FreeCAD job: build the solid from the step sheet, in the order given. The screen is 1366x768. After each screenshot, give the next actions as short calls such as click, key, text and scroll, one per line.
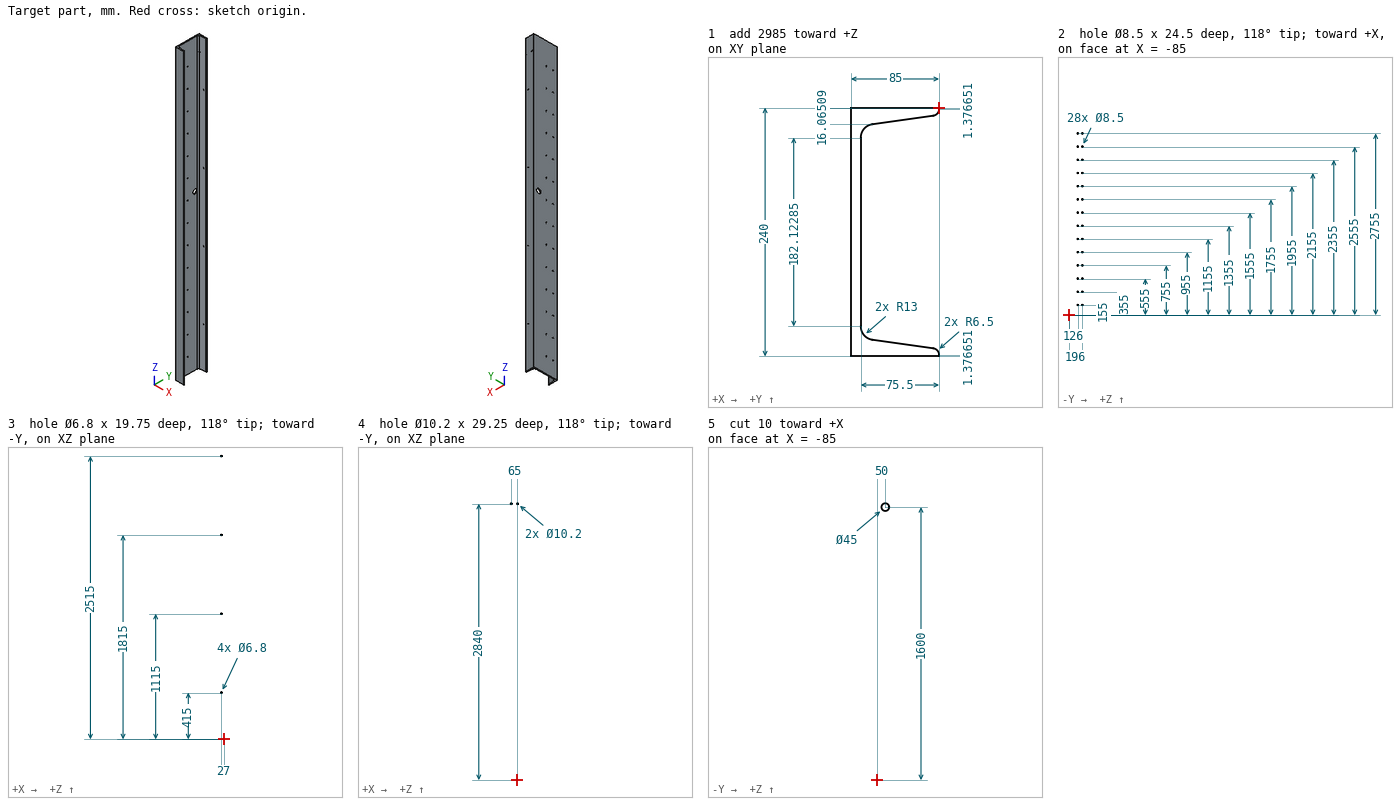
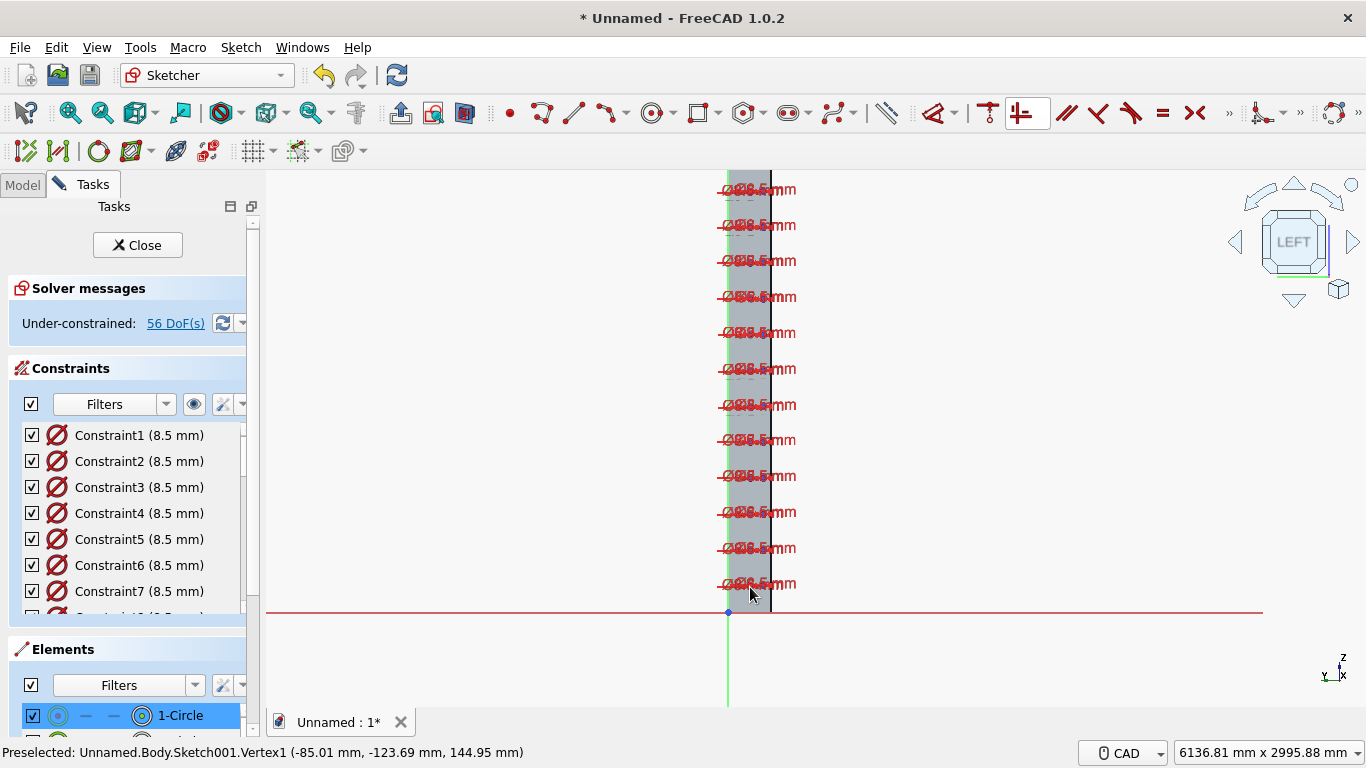
click(764, 585)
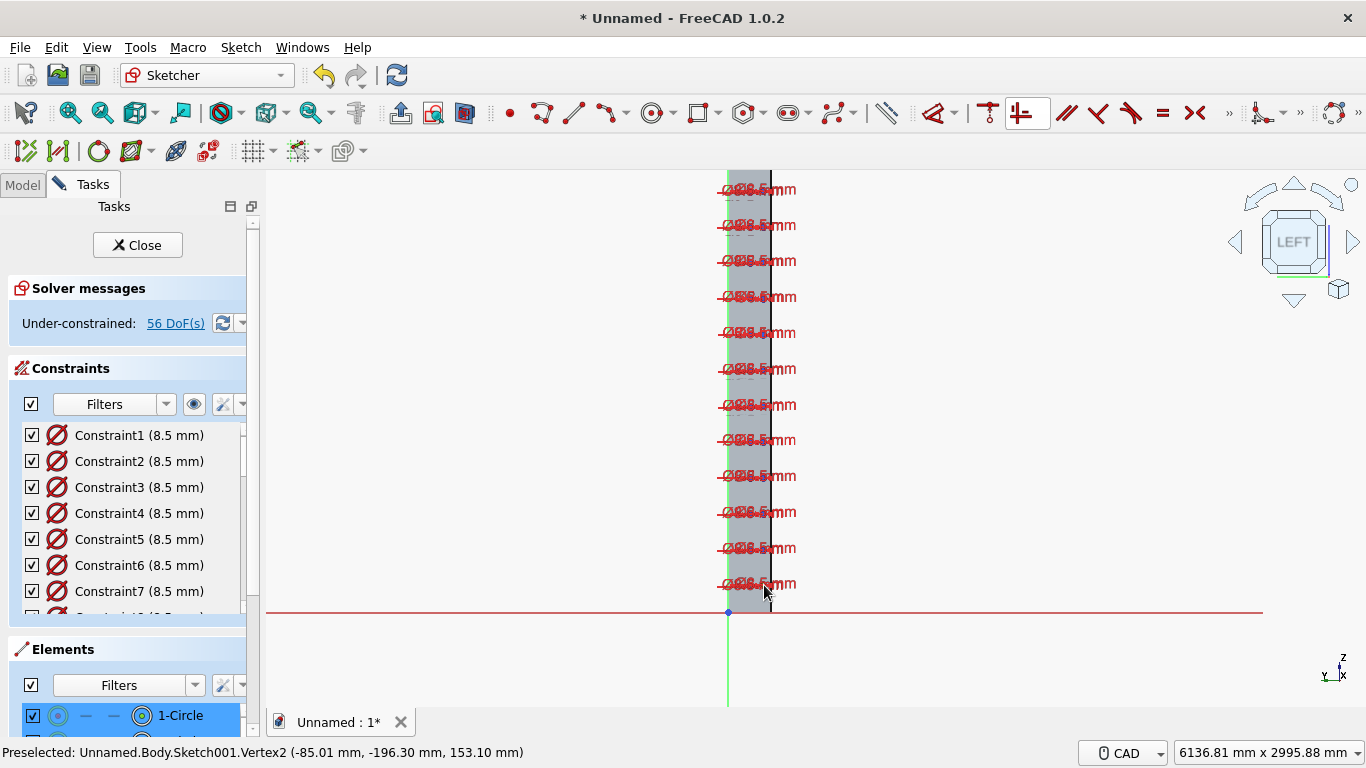
click(1044, 114)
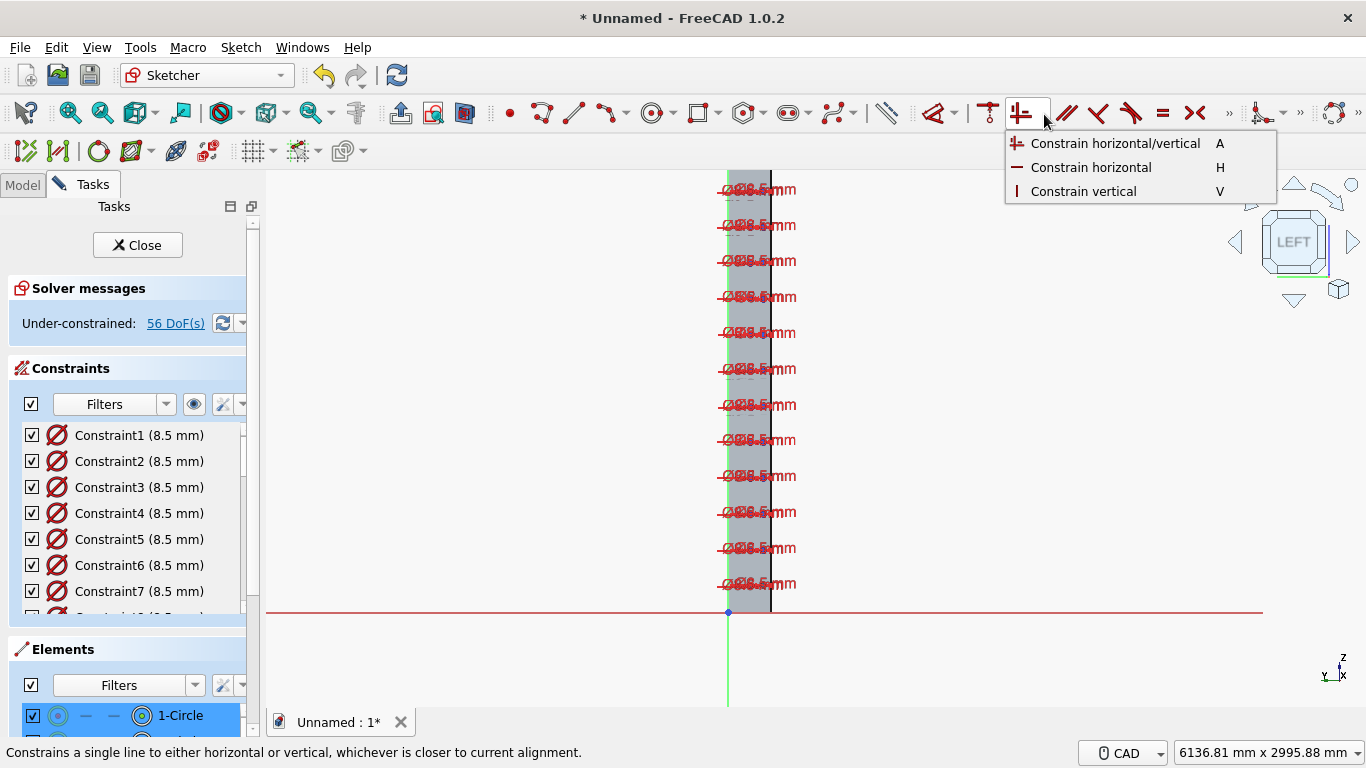
click(1141, 167)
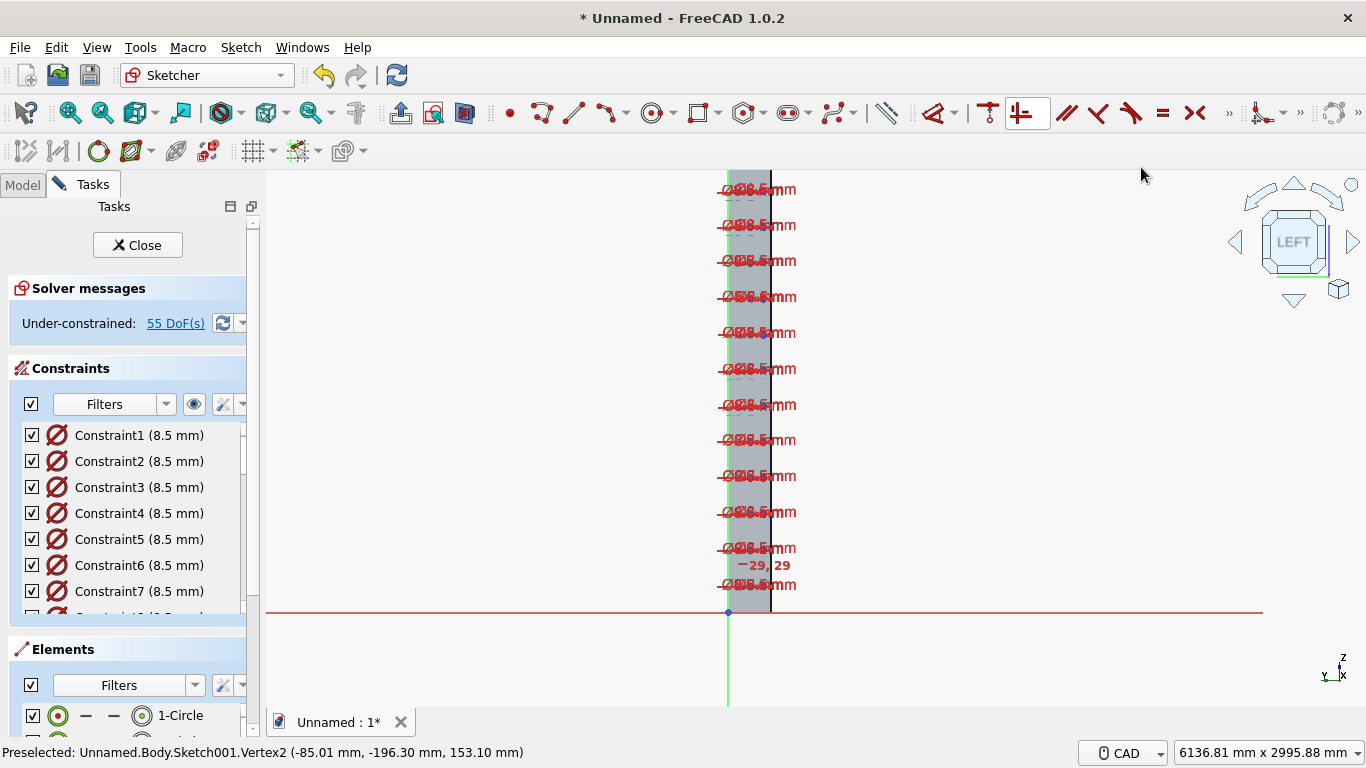
click(750, 587)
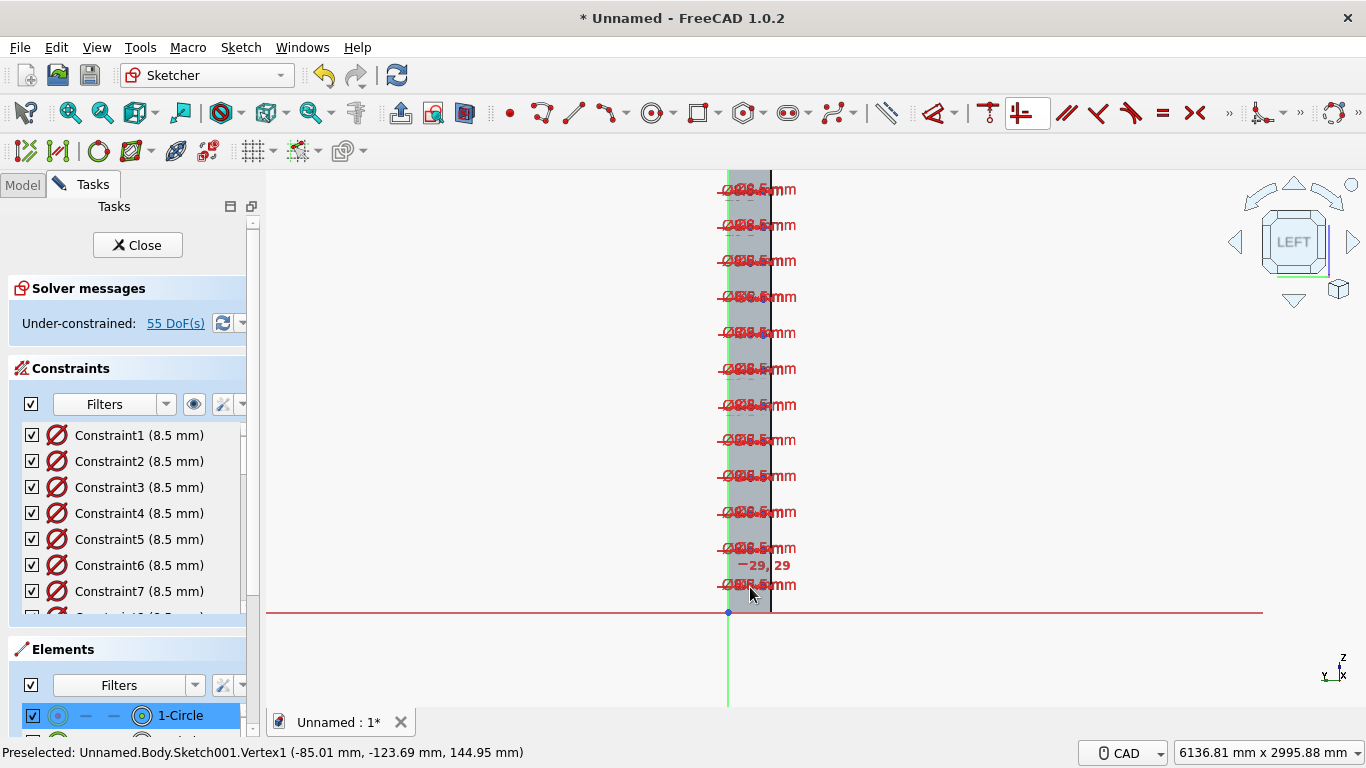
click(751, 551)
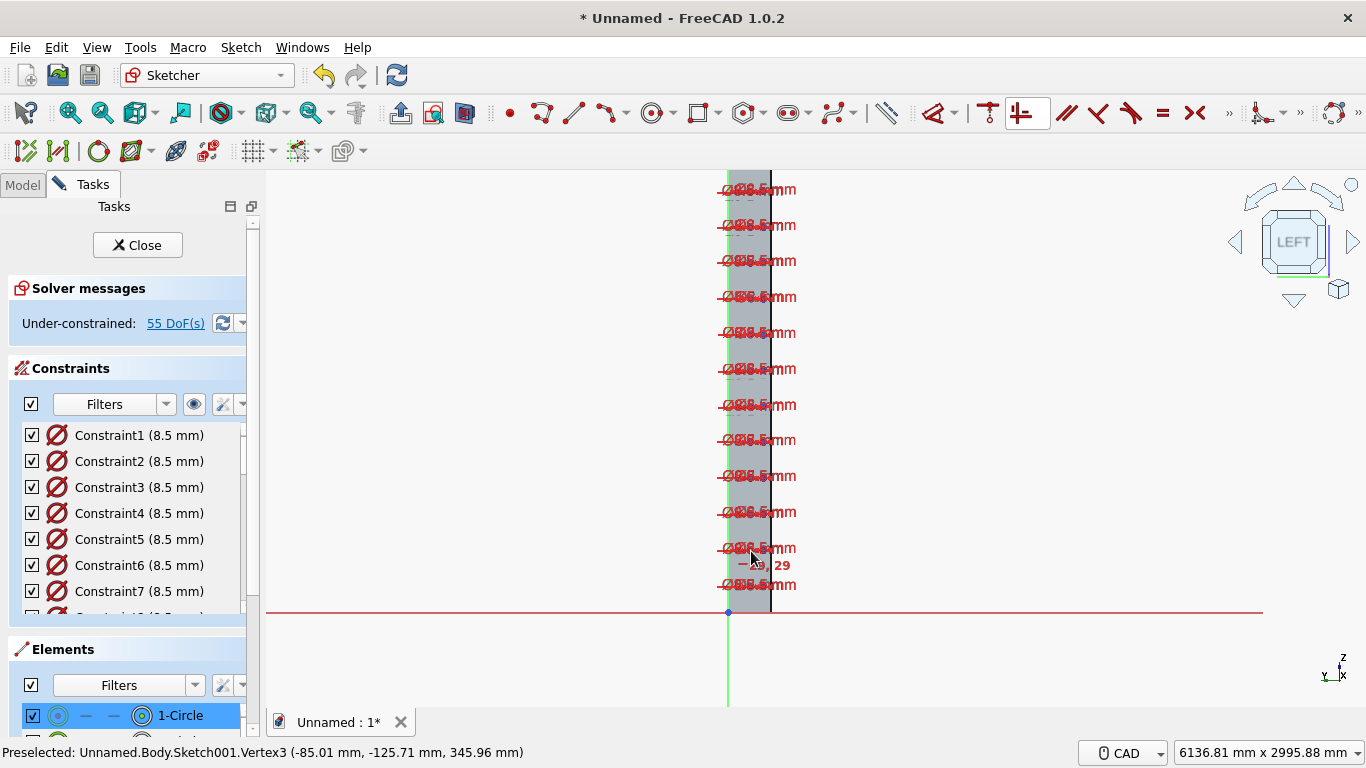
key(v)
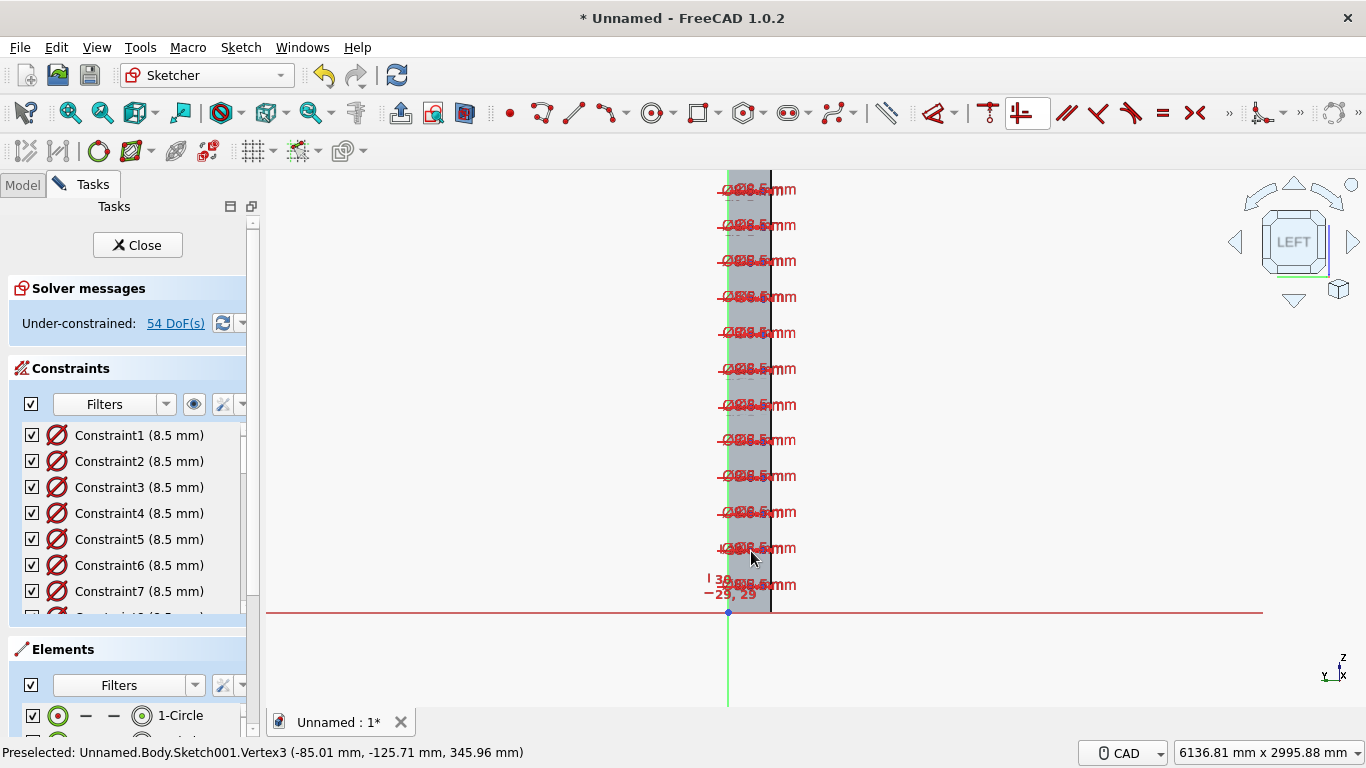
click(764, 587)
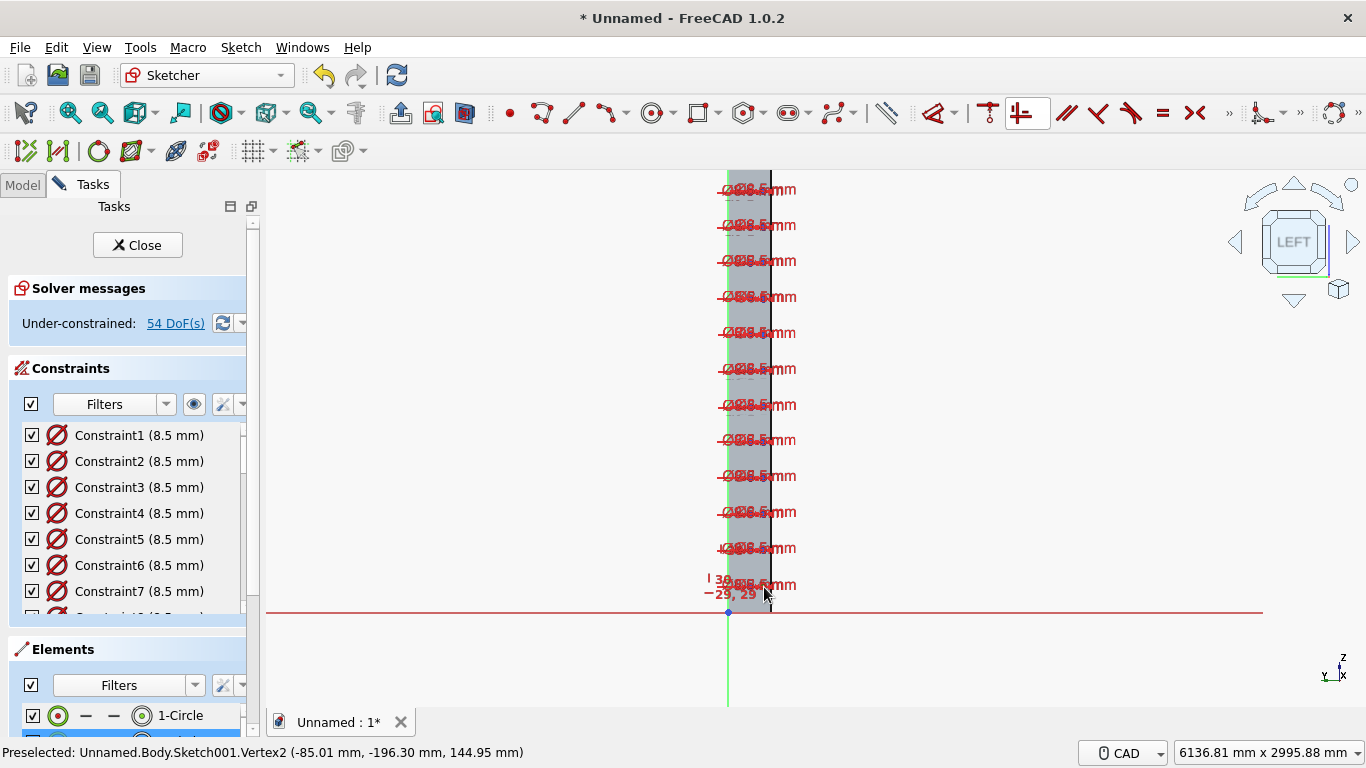
click(763, 550)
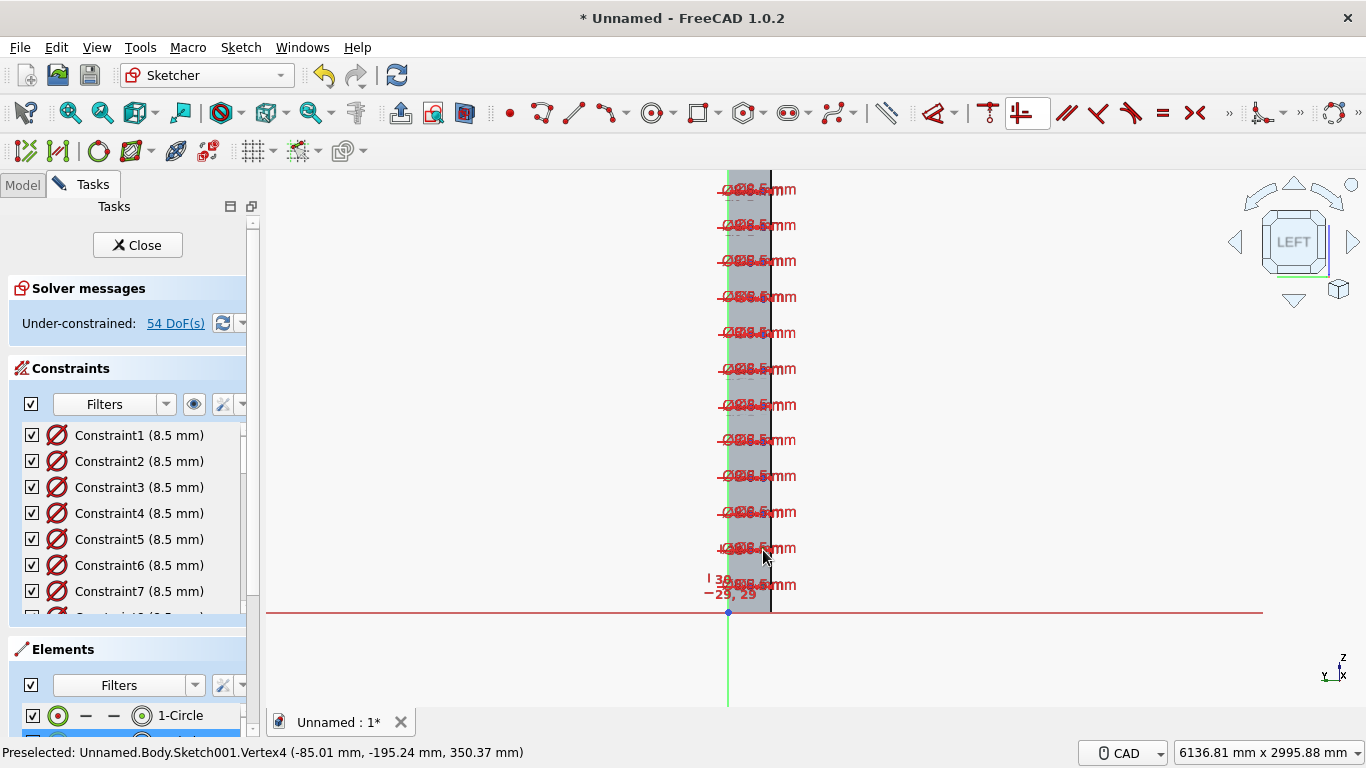
key(v)